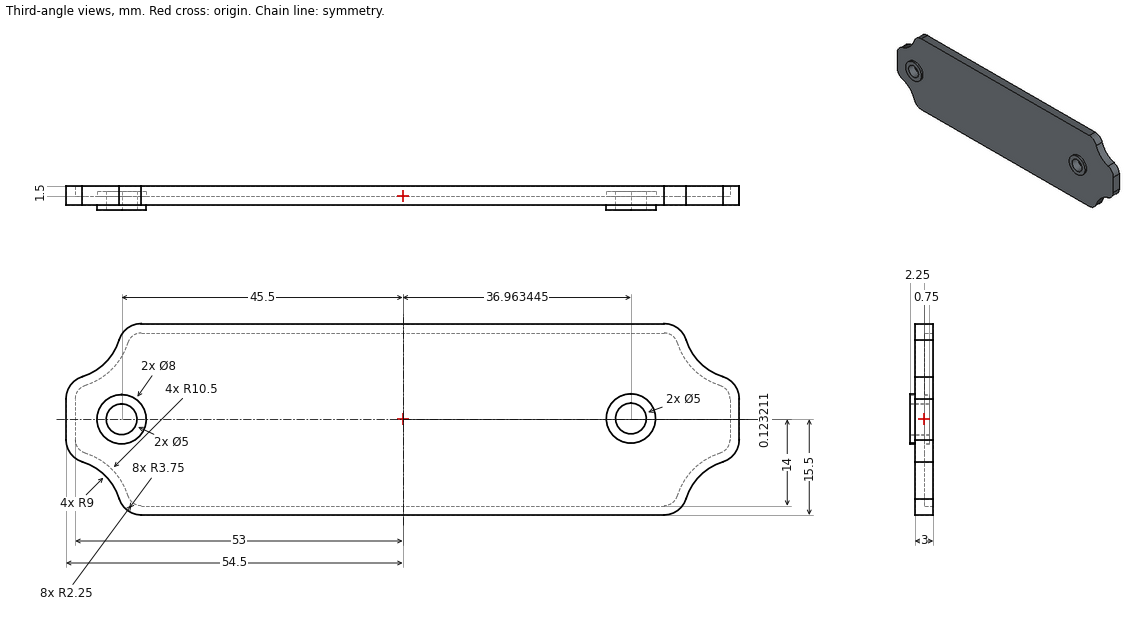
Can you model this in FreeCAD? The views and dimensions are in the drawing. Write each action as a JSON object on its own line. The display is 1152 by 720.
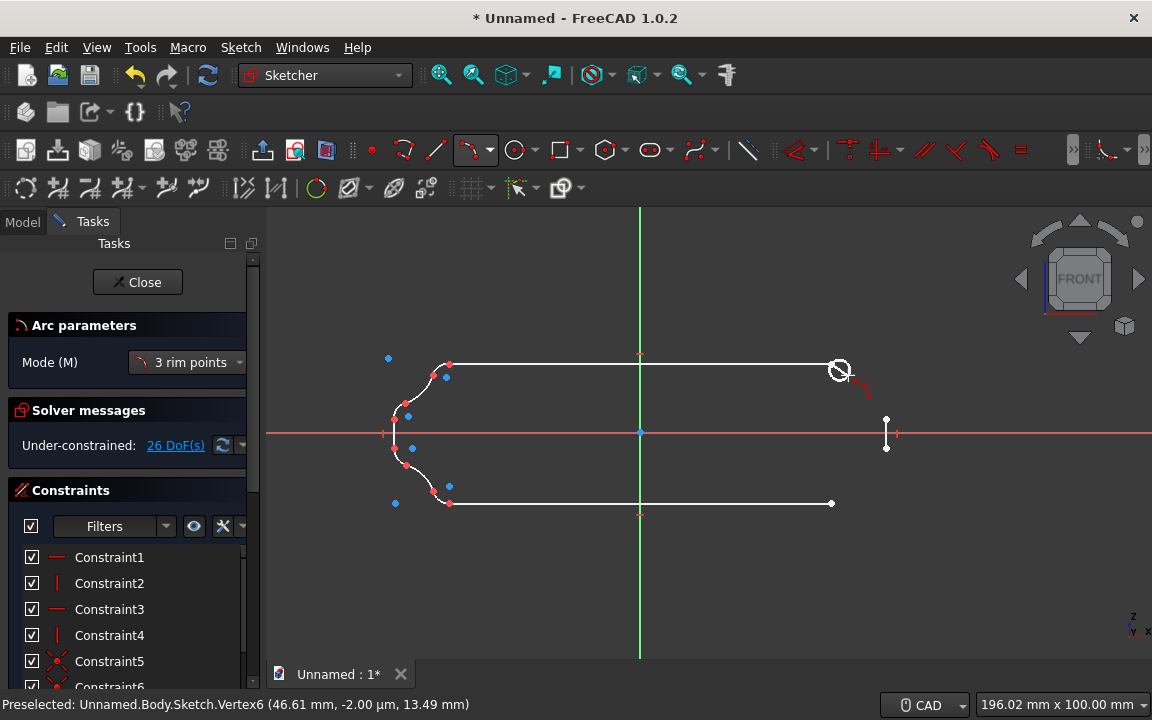
{"action": "scroll", "coordinate": [842, 366], "scroll_direction": "up", "scroll_amount": 8}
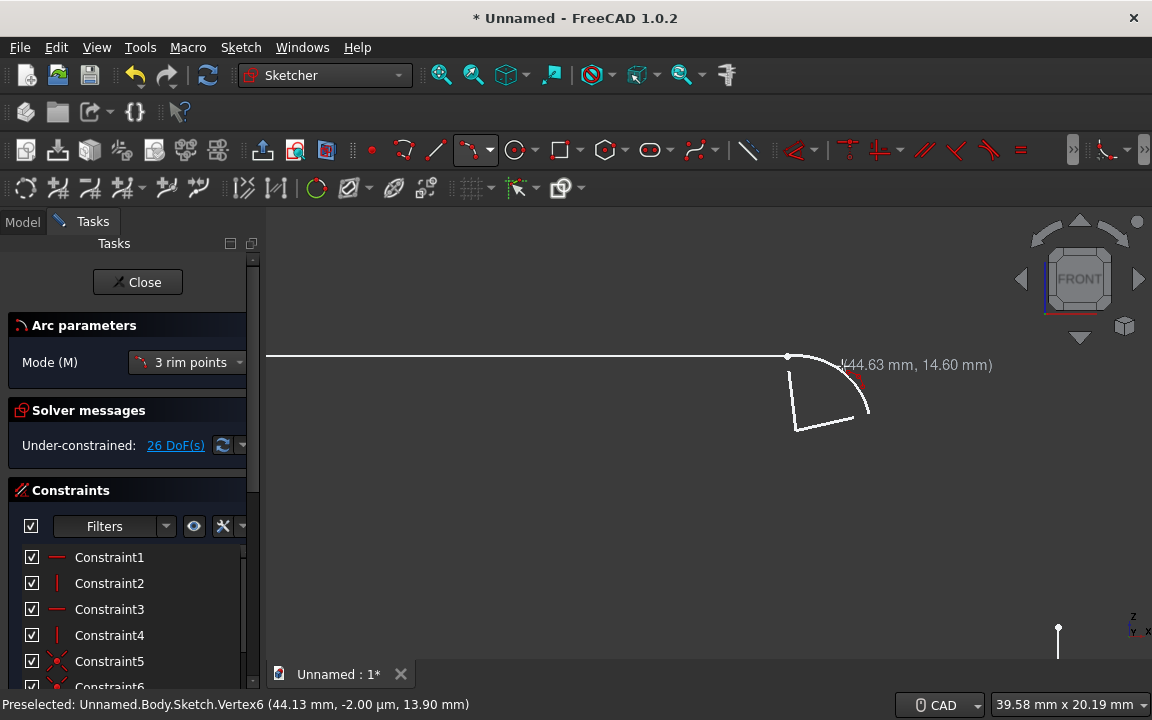
{"action": "left_click", "coordinate": [838, 366]}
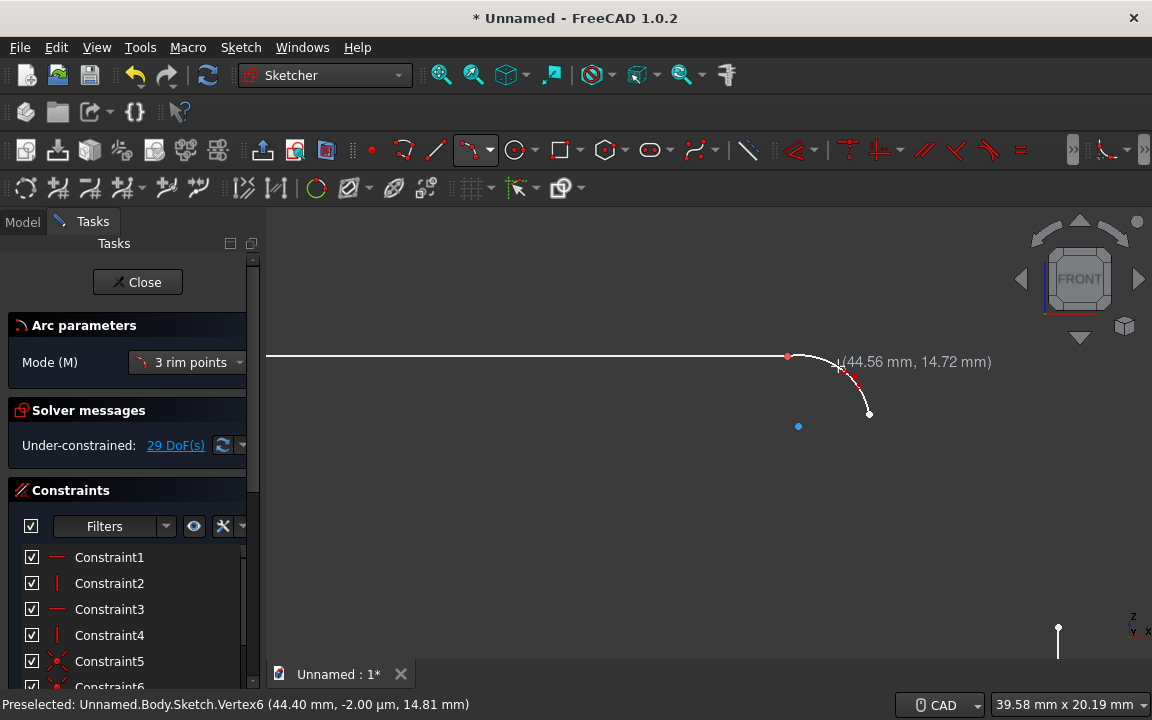
{"action": "scroll", "coordinate": [843, 366], "scroll_direction": "down", "scroll_amount": 8}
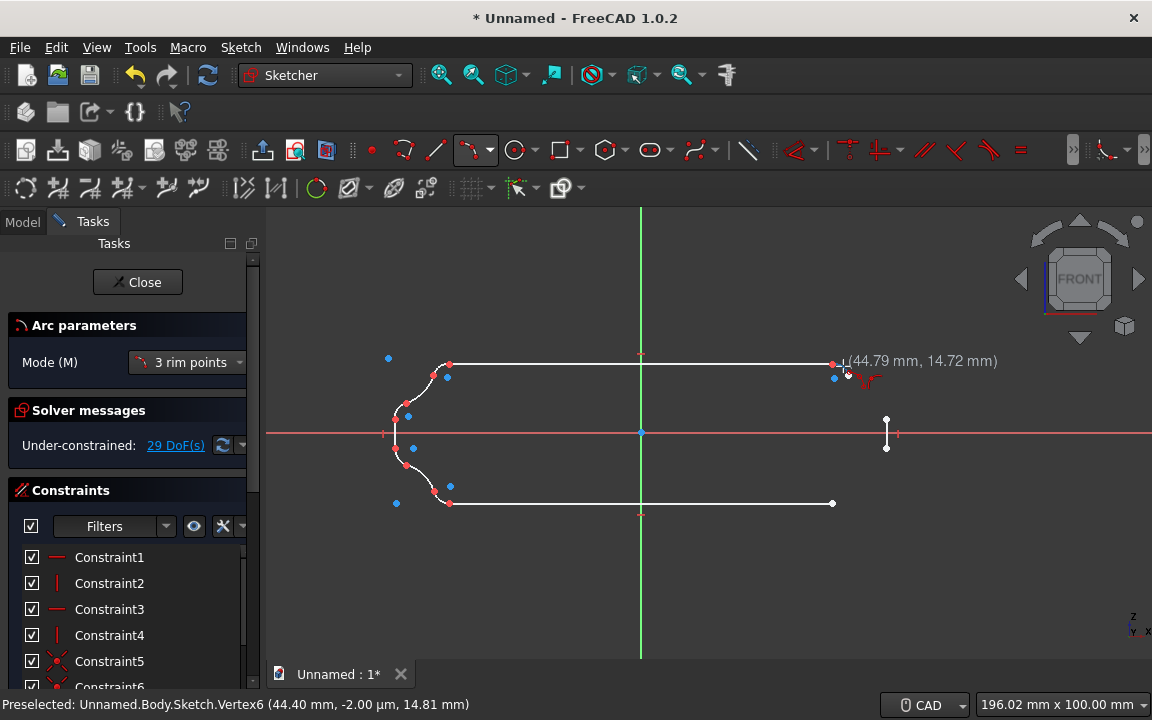
{"action": "left_click", "coordinate": [849, 376]}
{"action": "left_click", "coordinate": [875, 402]}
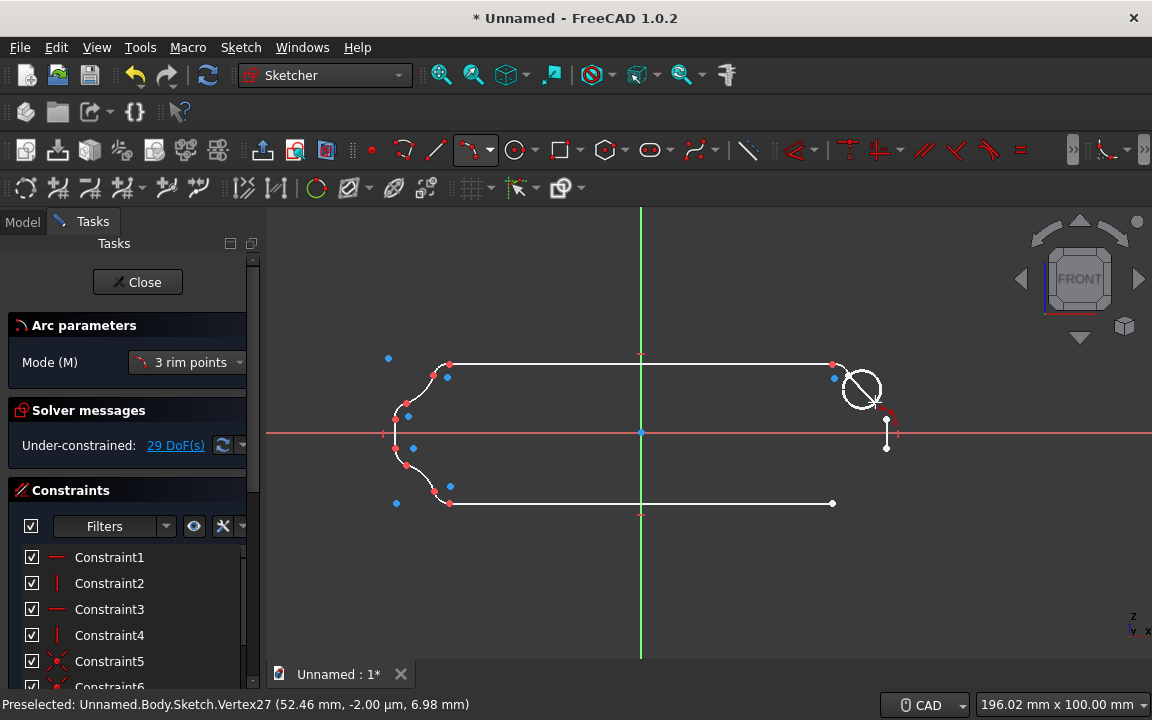
{"action": "scroll", "coordinate": [859, 392], "scroll_direction": "up", "scroll_amount": 7}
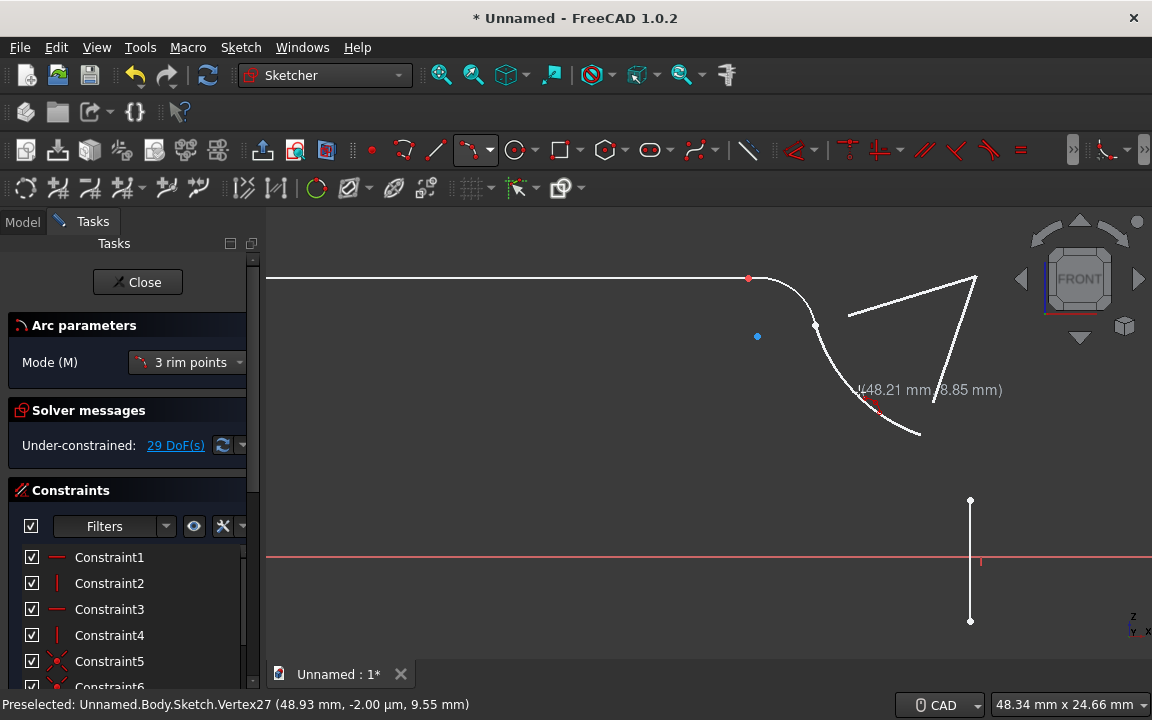
{"action": "left_click", "coordinate": [856, 390]}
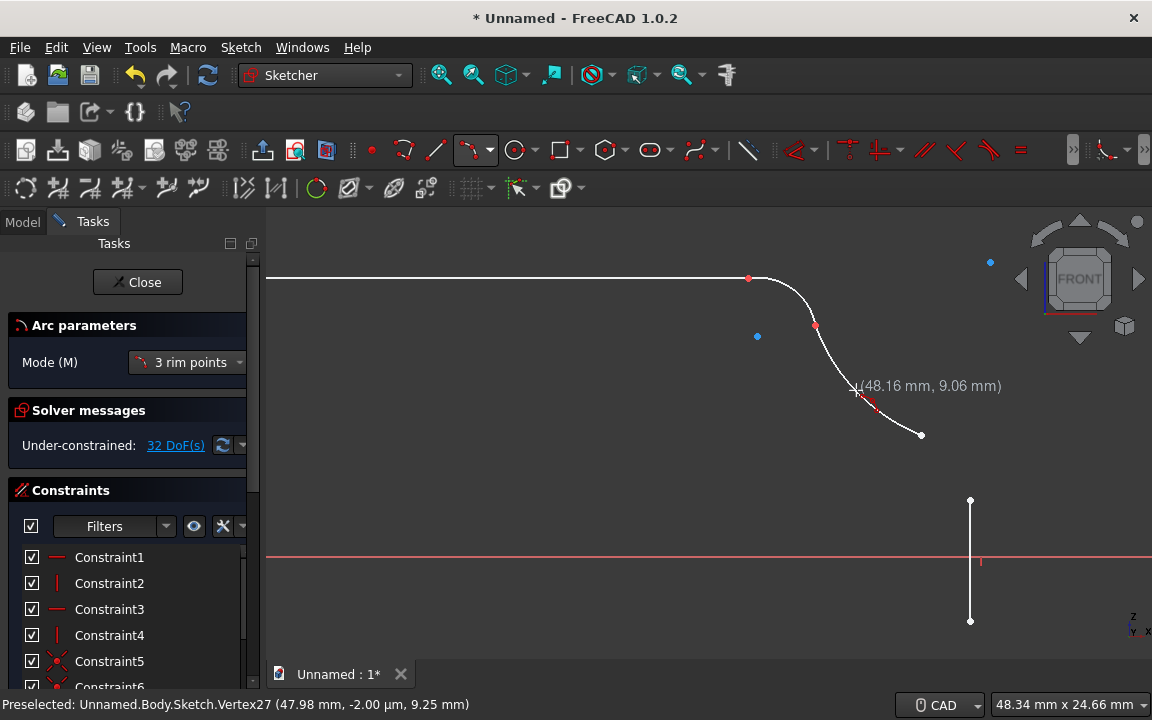
{"action": "scroll", "coordinate": [859, 392], "scroll_direction": "down", "scroll_amount": 7}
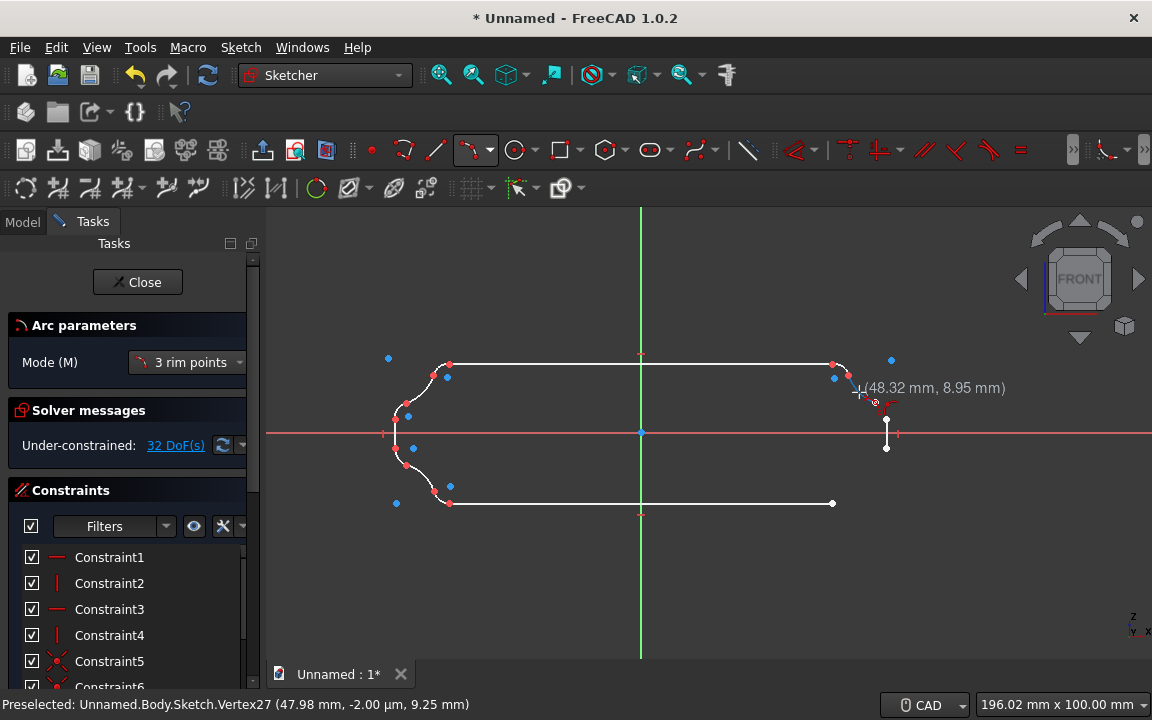
{"action": "left_click", "coordinate": [875, 403]}
{"action": "left_click", "coordinate": [887, 419]}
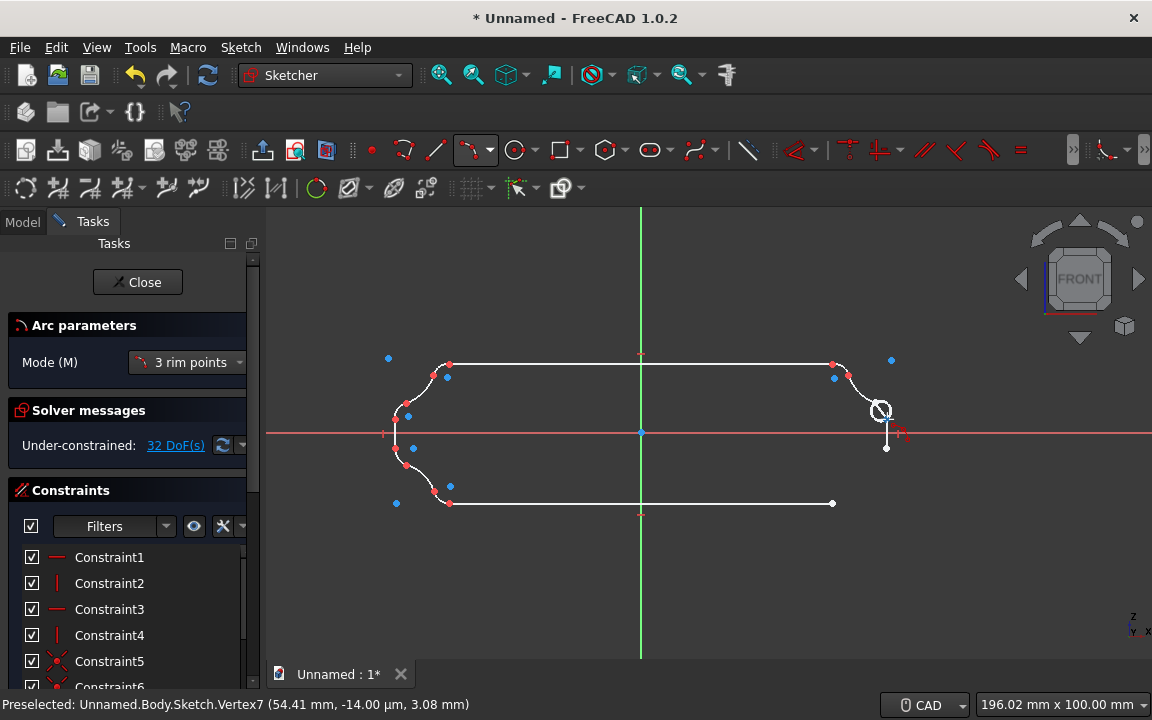
{"action": "scroll", "coordinate": [884, 408], "scroll_direction": "up", "scroll_amount": 8}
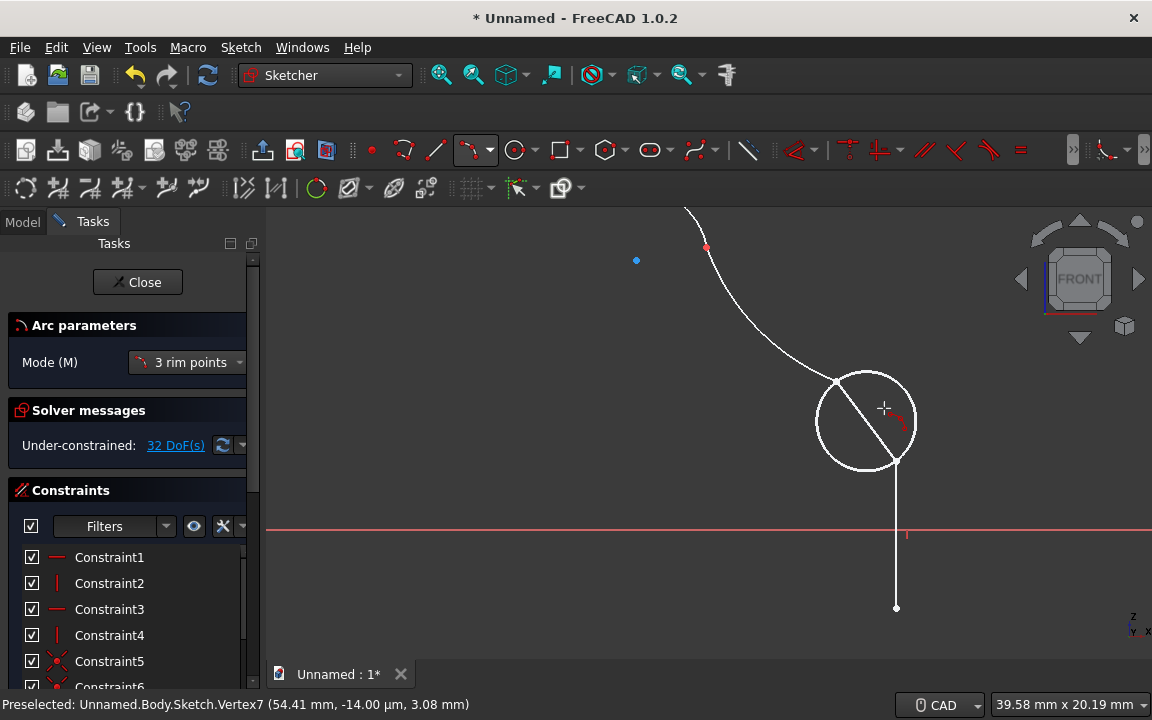
{"action": "left_click", "coordinate": [882, 406]}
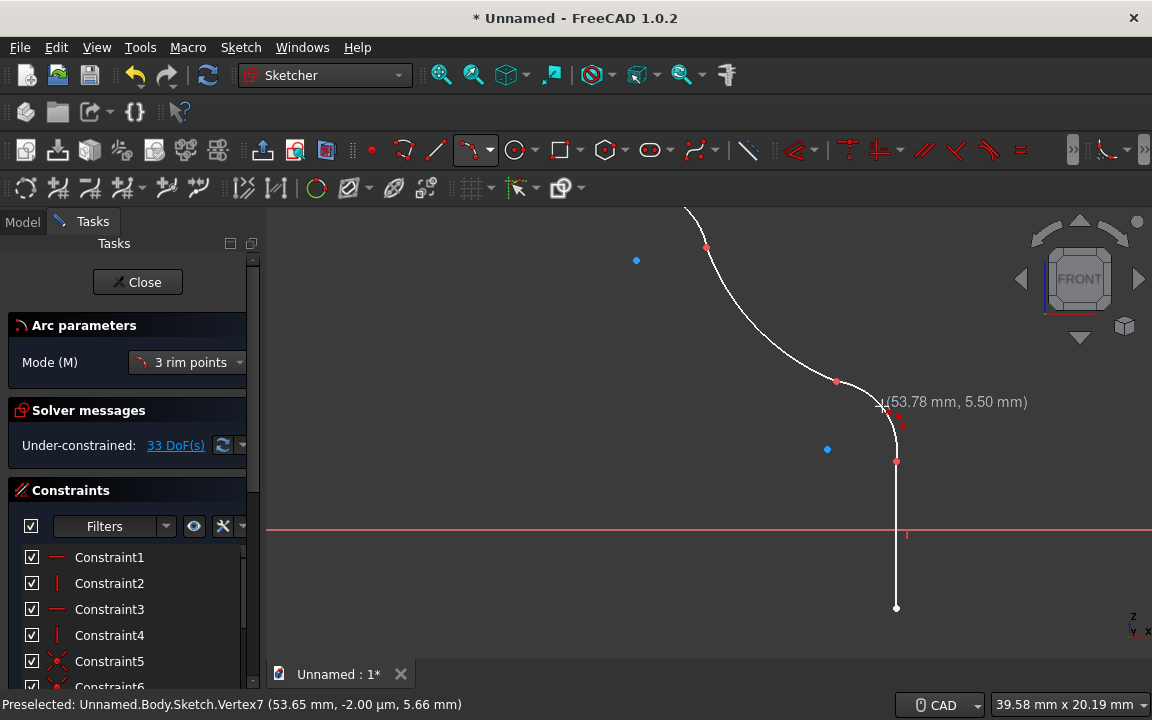
{"action": "scroll", "coordinate": [884, 408], "scroll_direction": "down", "scroll_amount": 8}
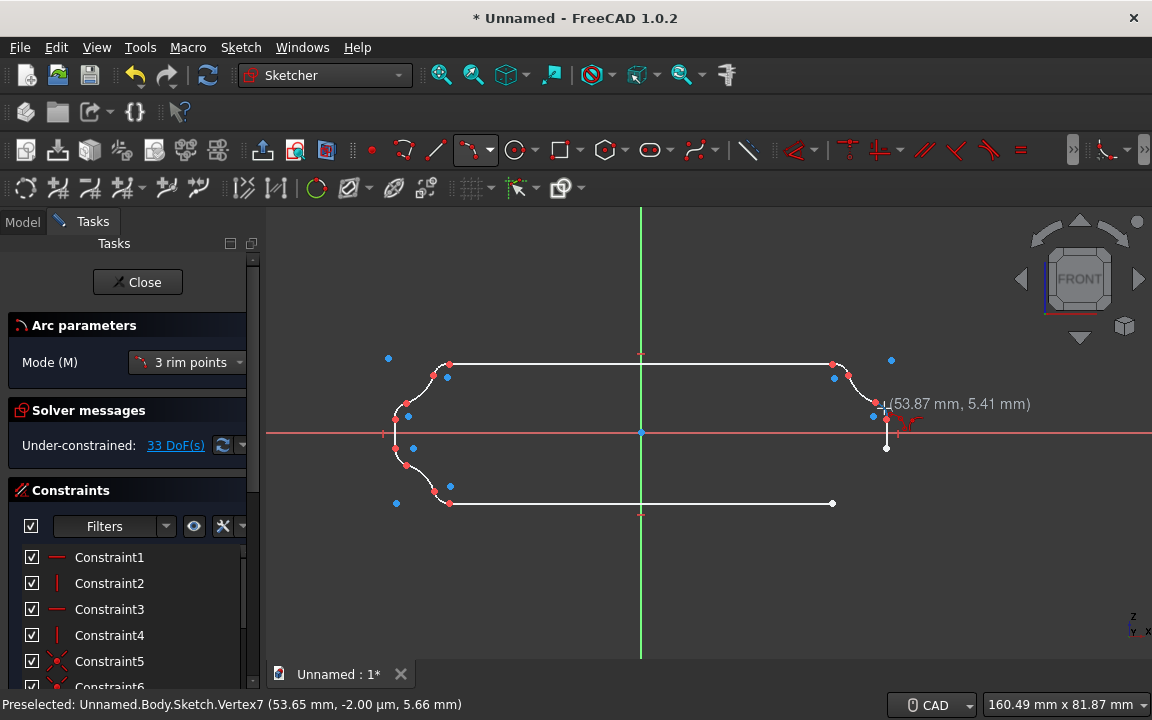
{"action": "left_click", "coordinate": [887, 449]}
{"action": "left_click", "coordinate": [875, 464]}